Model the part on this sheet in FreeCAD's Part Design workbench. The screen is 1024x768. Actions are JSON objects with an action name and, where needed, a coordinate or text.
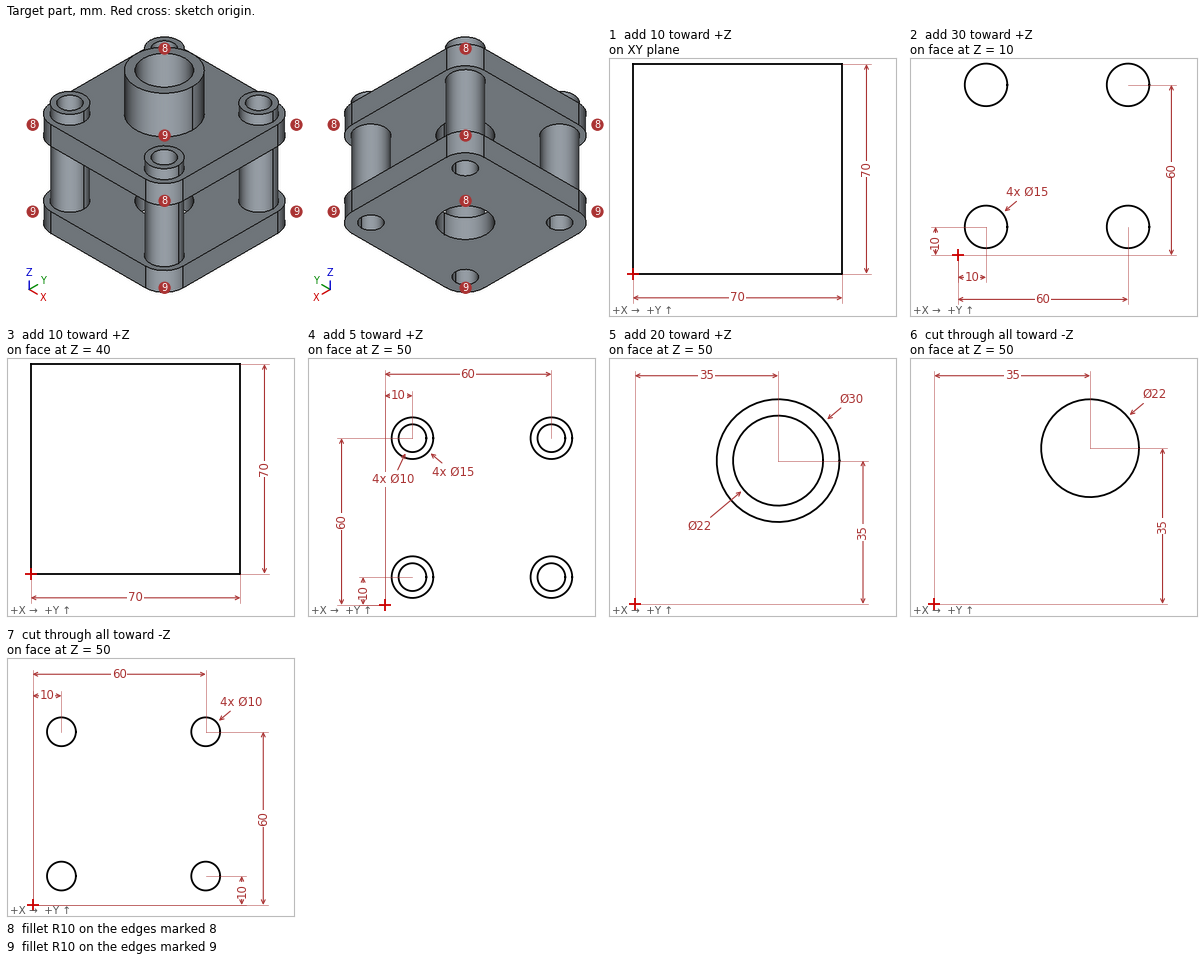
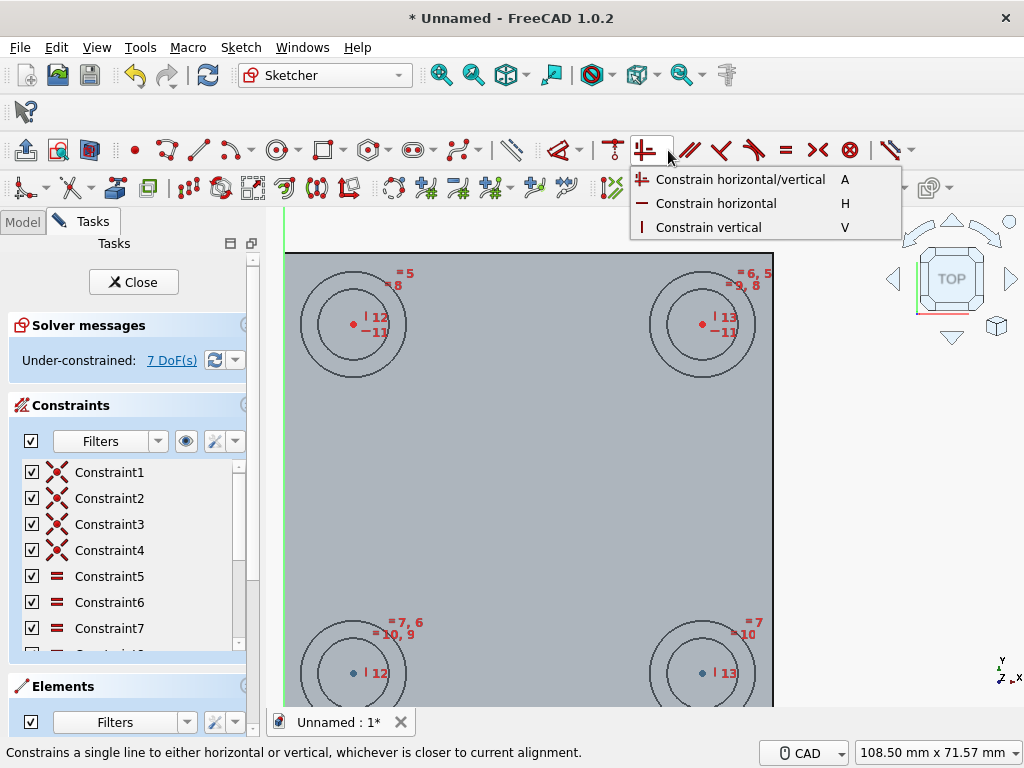
{"action": "left_click", "coordinate": [766, 203]}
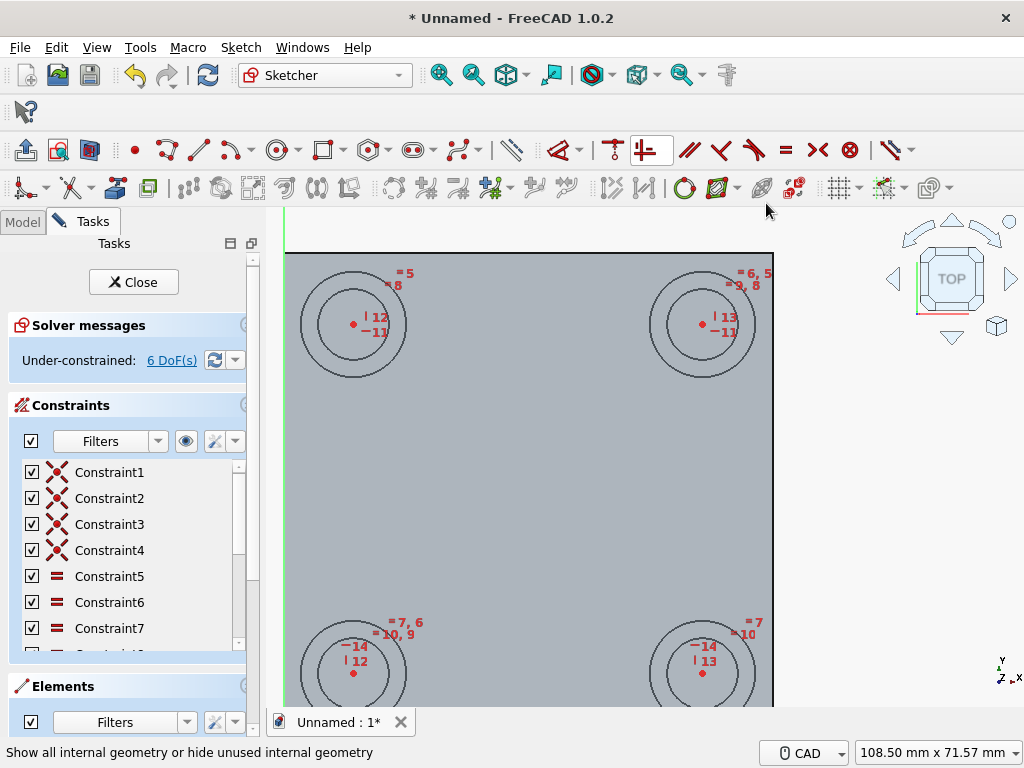
{"action": "key", "text": "d"}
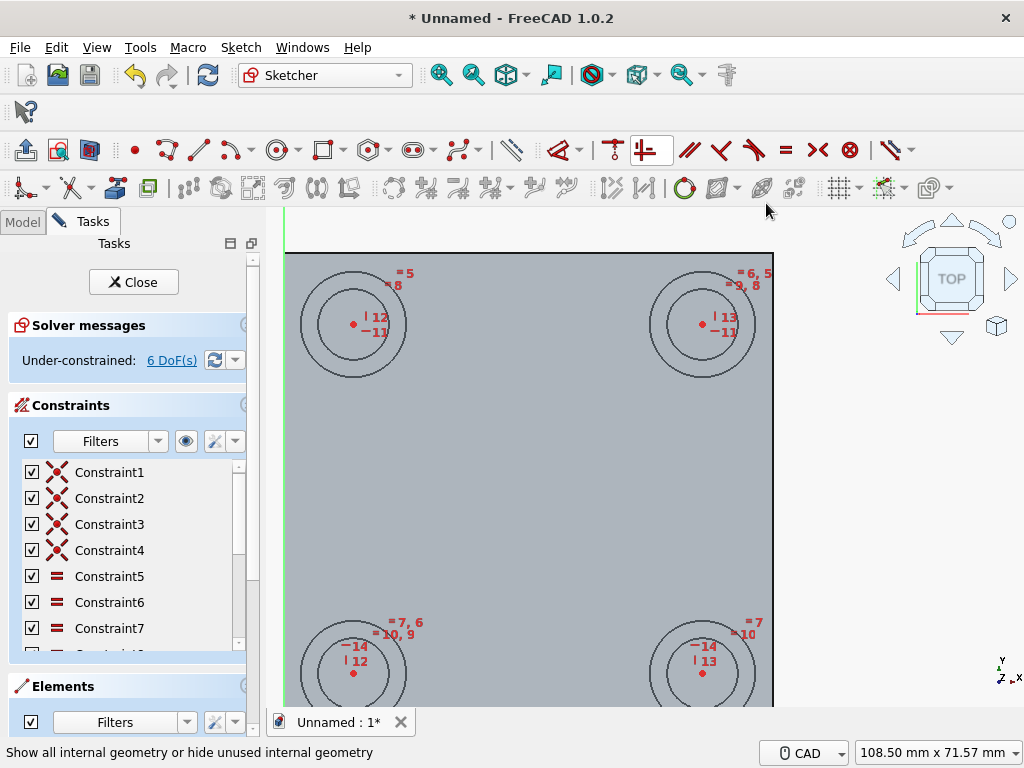
{"action": "left_click", "coordinate": [391, 287]}
{"action": "left_click", "coordinate": [414, 264]}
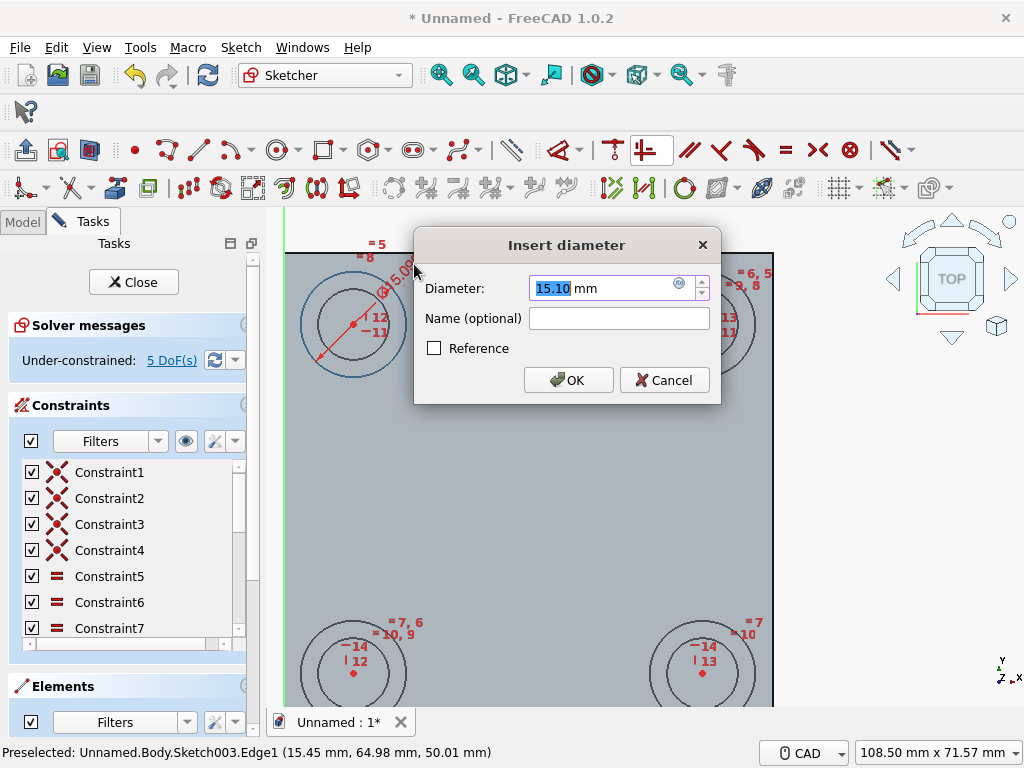
{"action": "type", "text": "15"}
{"action": "key", "text": "Return"}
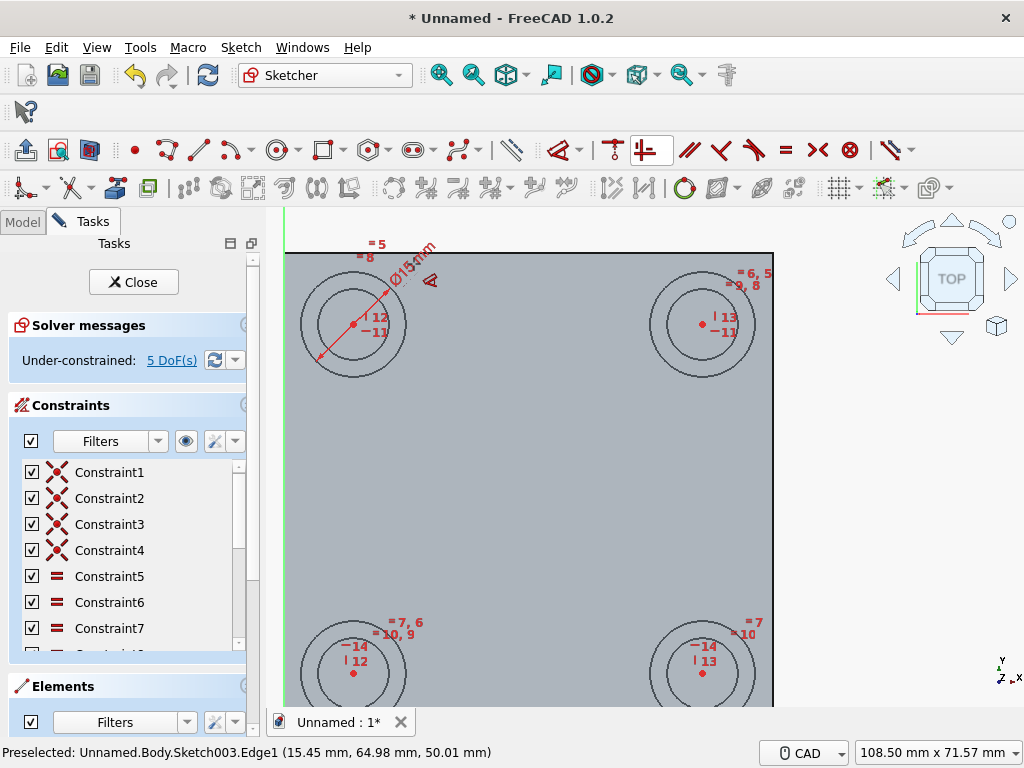
{"action": "left_click", "coordinate": [378, 299]}
{"action": "left_click", "coordinate": [418, 304]}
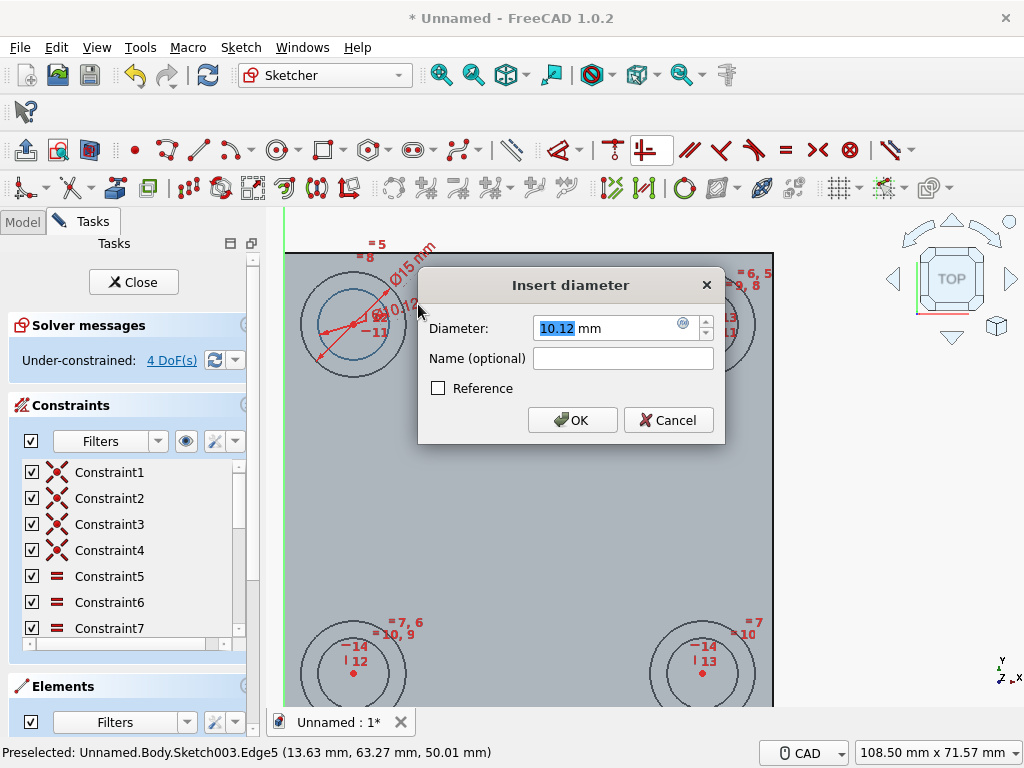
{"action": "type", "text": "10"}
{"action": "key", "text": "Return"}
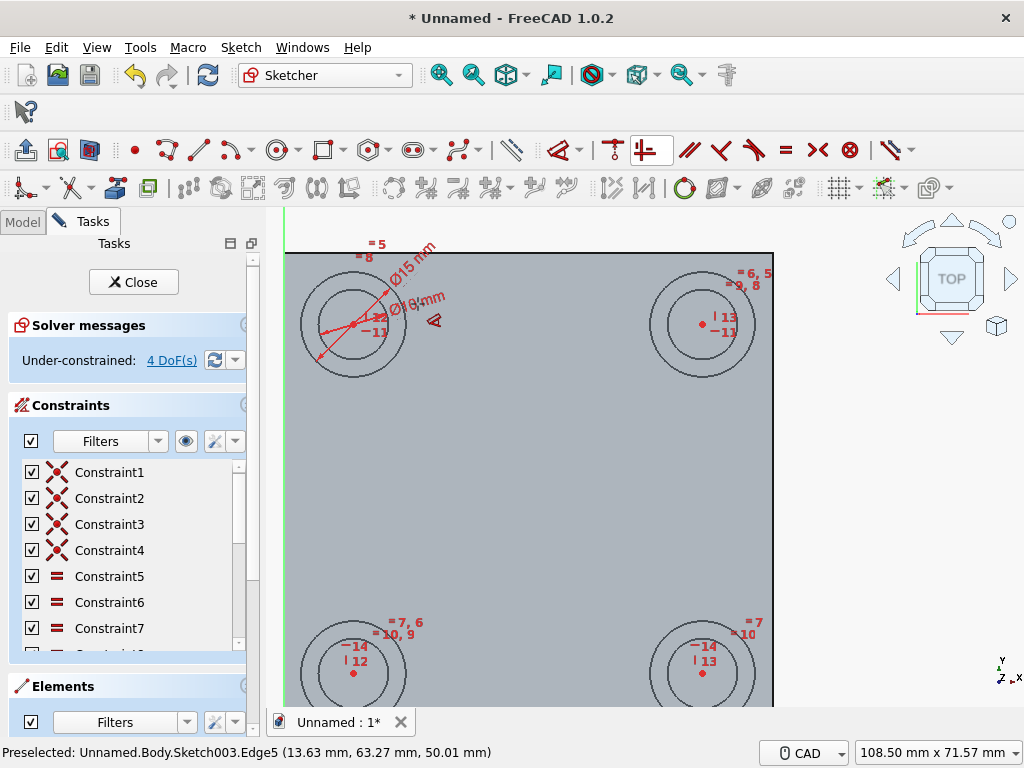
{"action": "left_click", "coordinate": [353, 324]}
{"action": "left_click", "coordinate": [310, 266]}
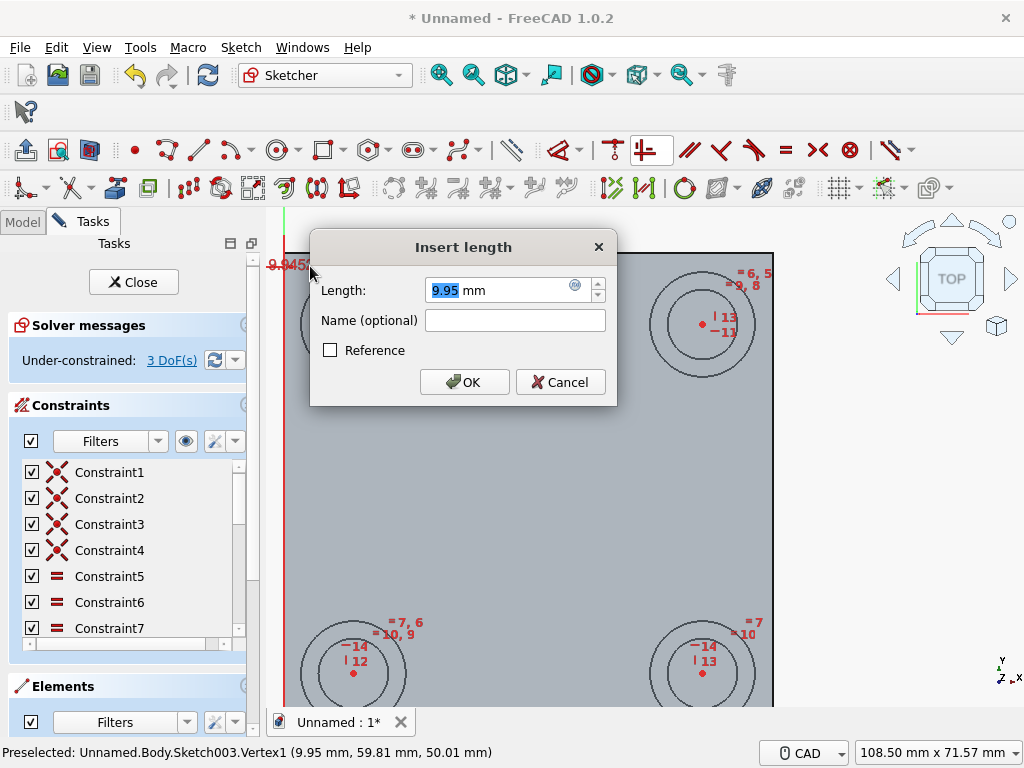
{"action": "type", "text": "10"}
{"action": "key", "text": "Return"}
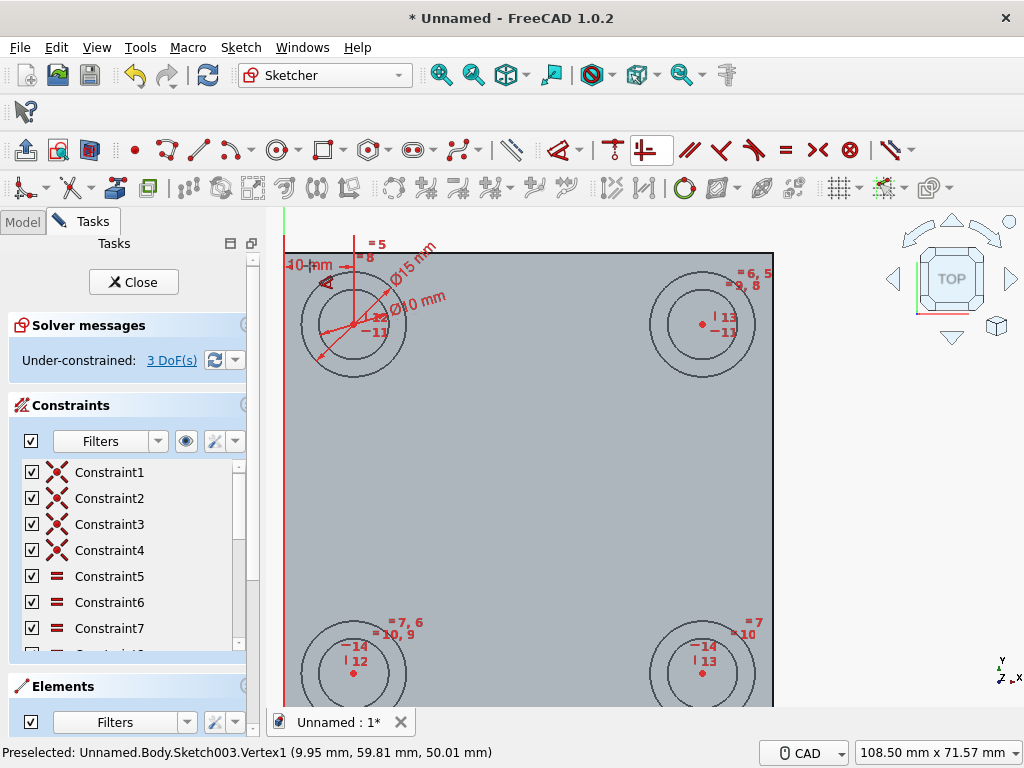
{"action": "left_click", "coordinate": [354, 324]}
{"action": "left_click", "coordinate": [388, 502]}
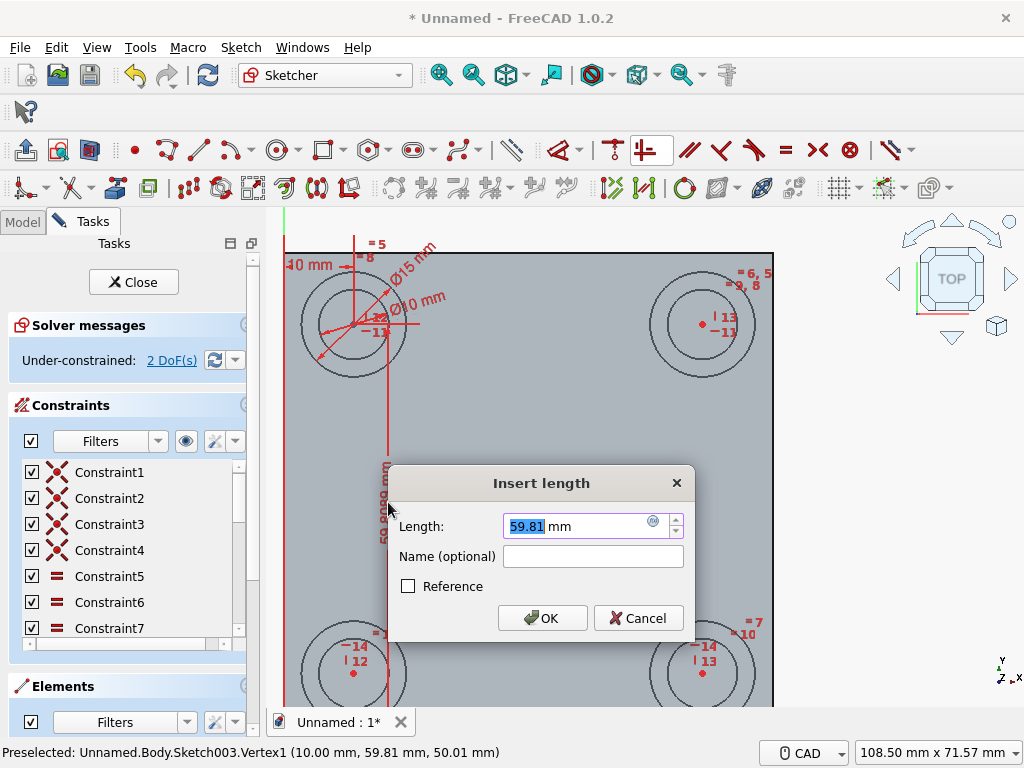
{"action": "type", "text": "60"}
{"action": "key", "text": "Return"}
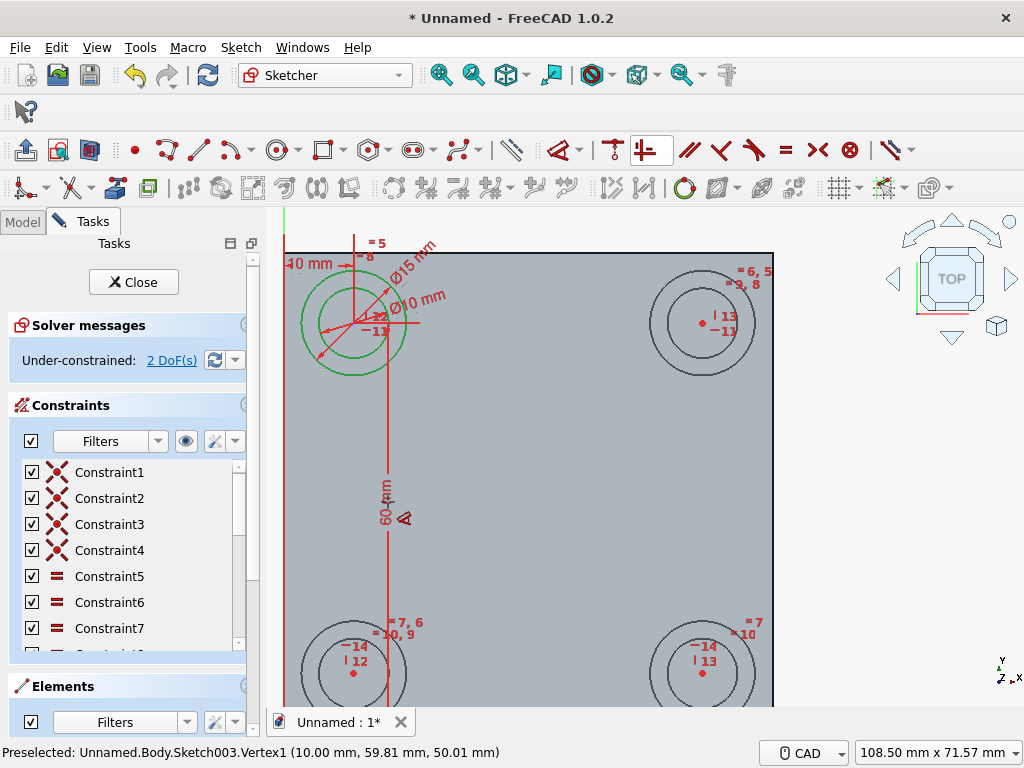
{"action": "left_click", "coordinate": [702, 323]}
{"action": "left_click", "coordinate": [498, 289]}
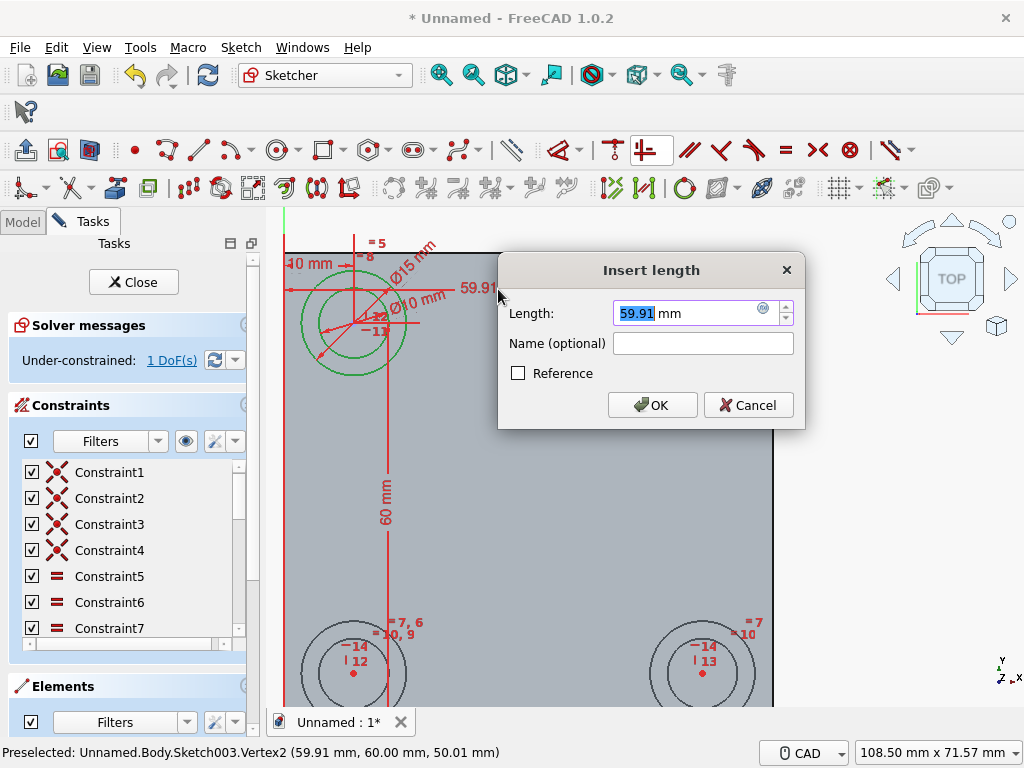
{"action": "type", "text": "60"}
{"action": "key", "text": "Return"}